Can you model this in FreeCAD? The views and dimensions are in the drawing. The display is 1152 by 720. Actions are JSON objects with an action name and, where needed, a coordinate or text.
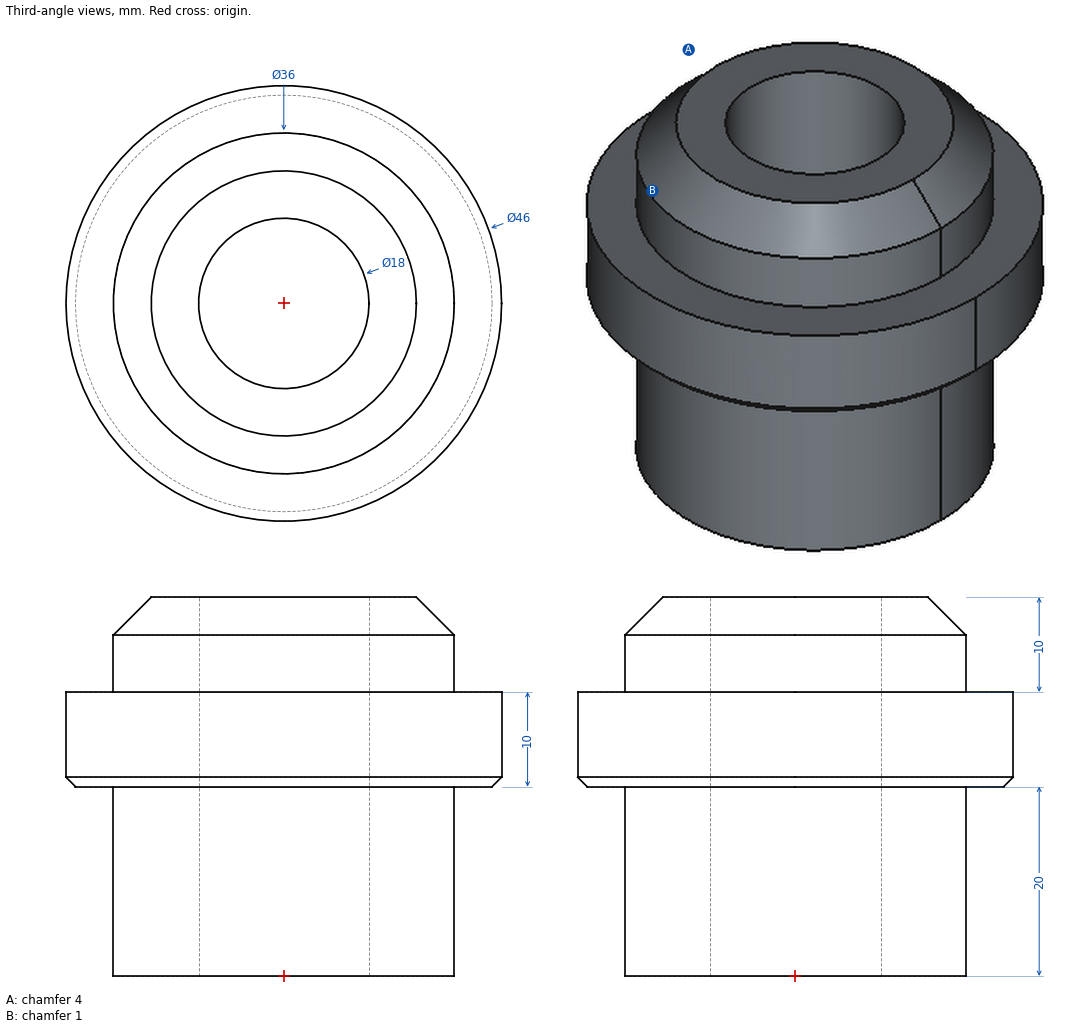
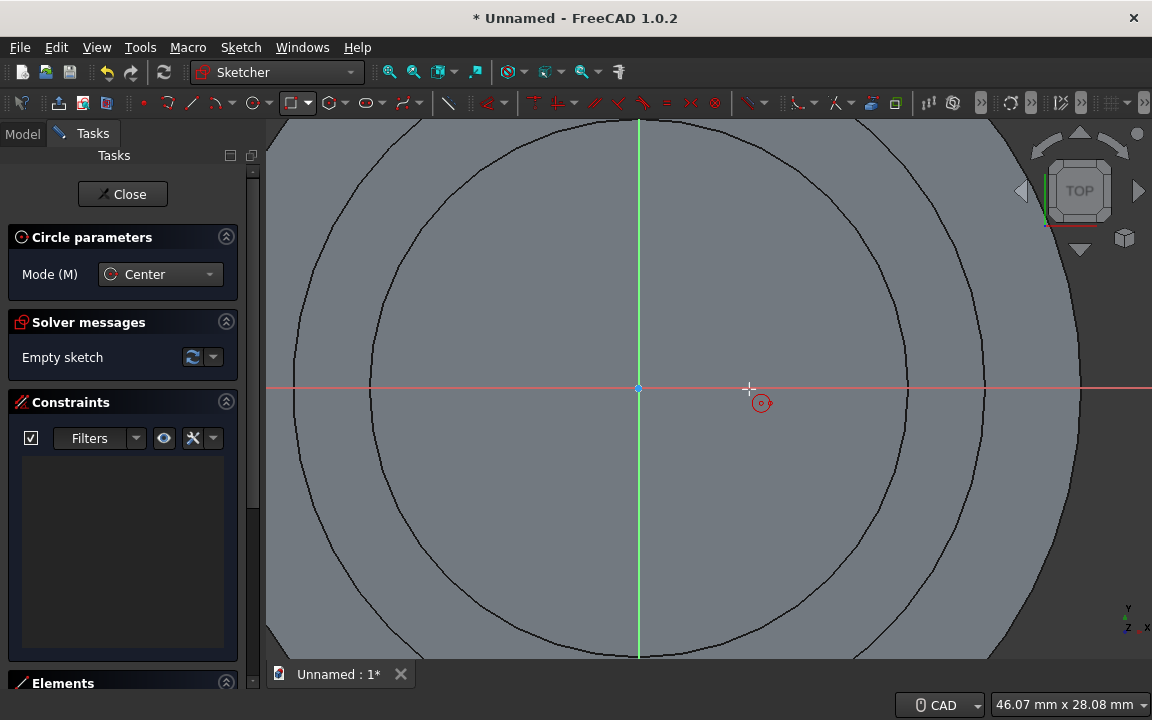
{"action": "left_click", "coordinate": [639, 388]}
{"action": "left_click", "coordinate": [761, 266]}
{"action": "key", "text": "Escape"}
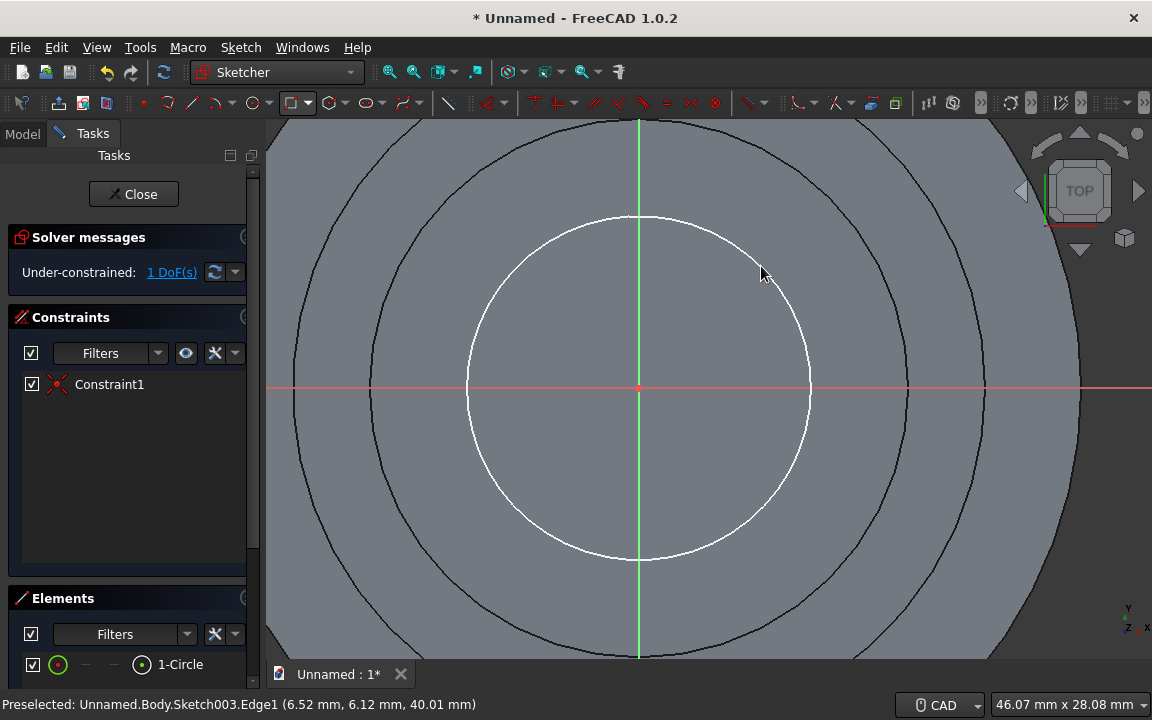
{"action": "left_click", "coordinate": [488, 104]}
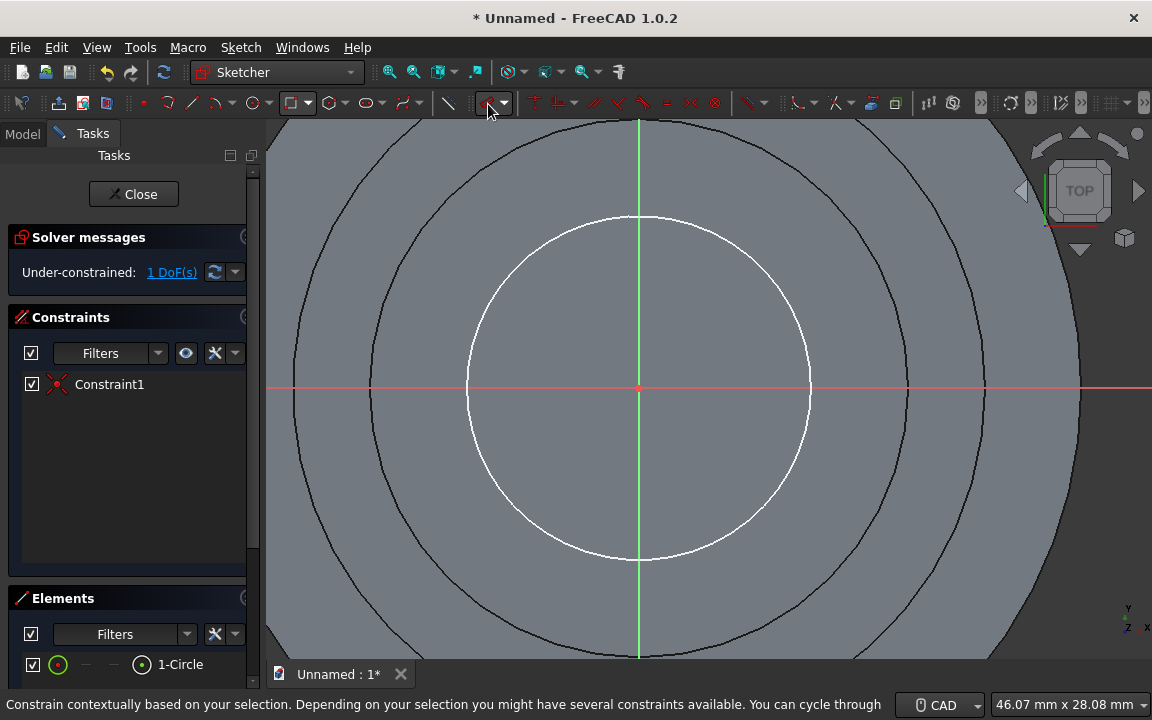
{"action": "left_click", "coordinate": [760, 266]}
{"action": "left_click", "coordinate": [783, 243]}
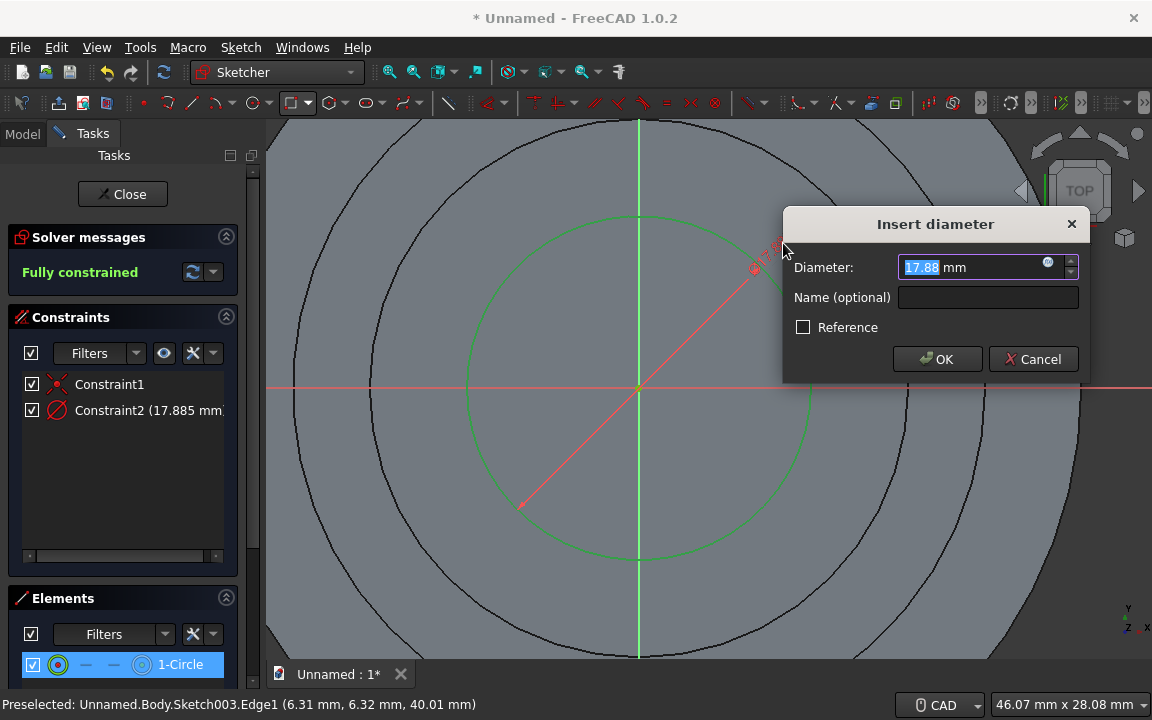
{"action": "type", "text": "18"}
{"action": "key", "text": "Return"}
{"action": "key", "text": "Escape"}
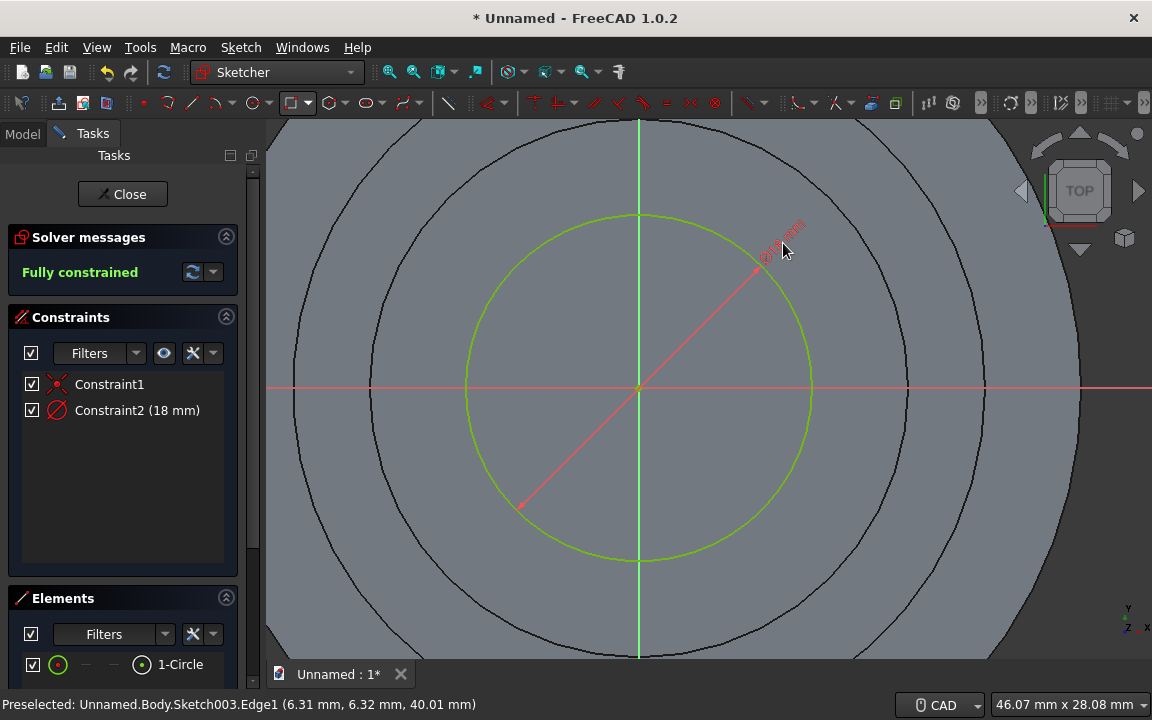
{"action": "left_click", "coordinate": [123, 194]}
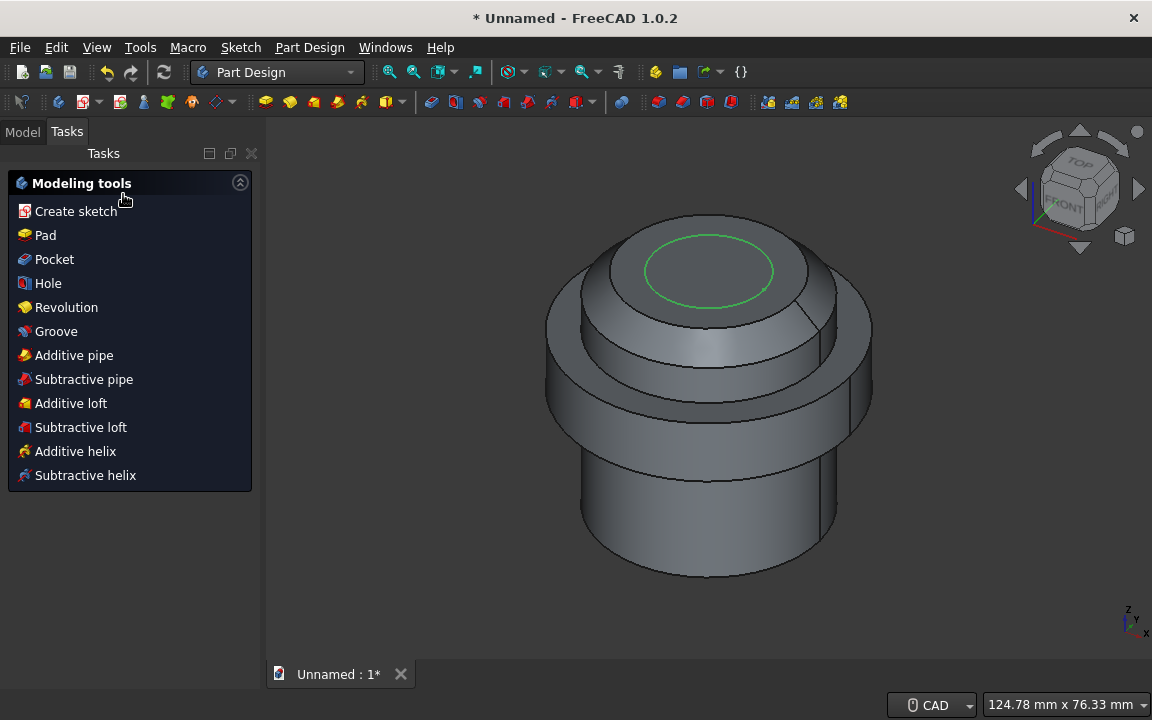
{"action": "left_click", "coordinate": [432, 102]}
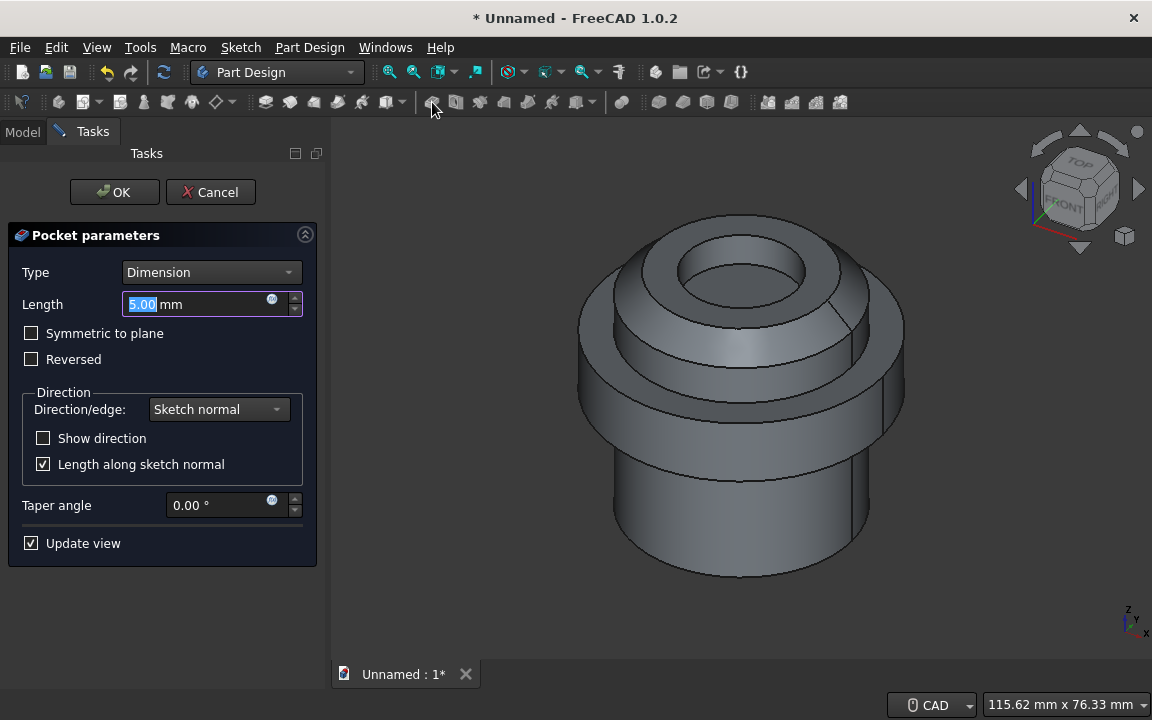
{"action": "left_click", "coordinate": [212, 272]}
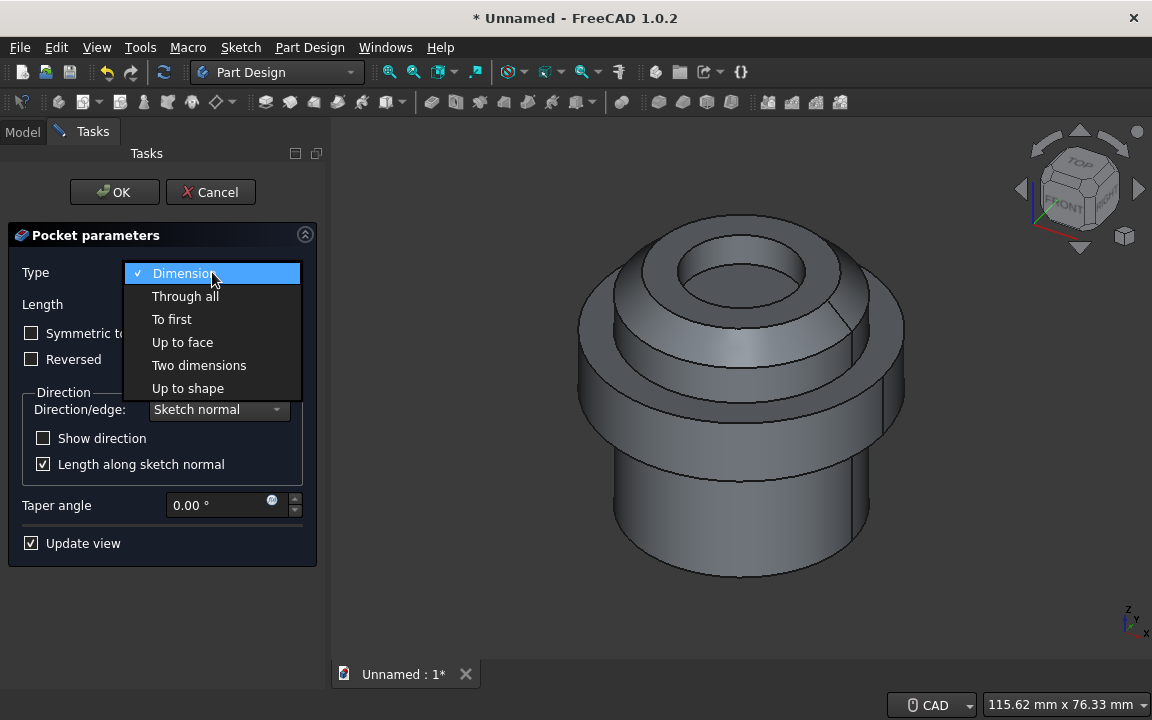
{"action": "left_click", "coordinate": [212, 296]}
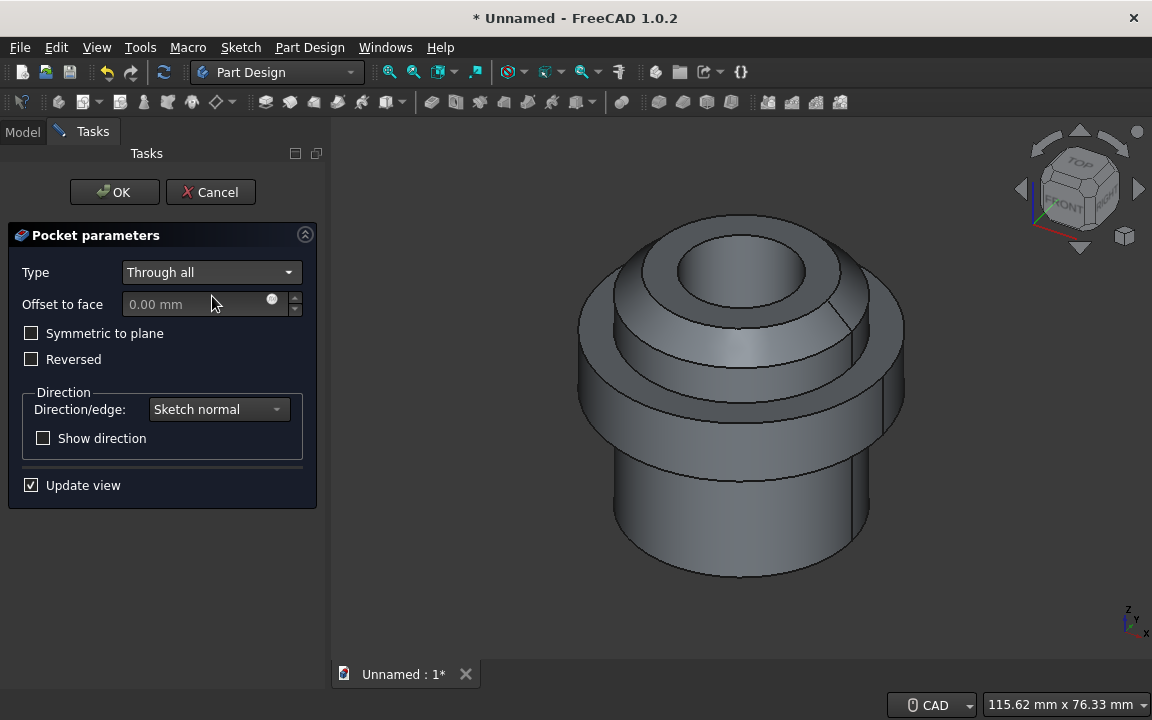
{"action": "left_click", "coordinate": [115, 192]}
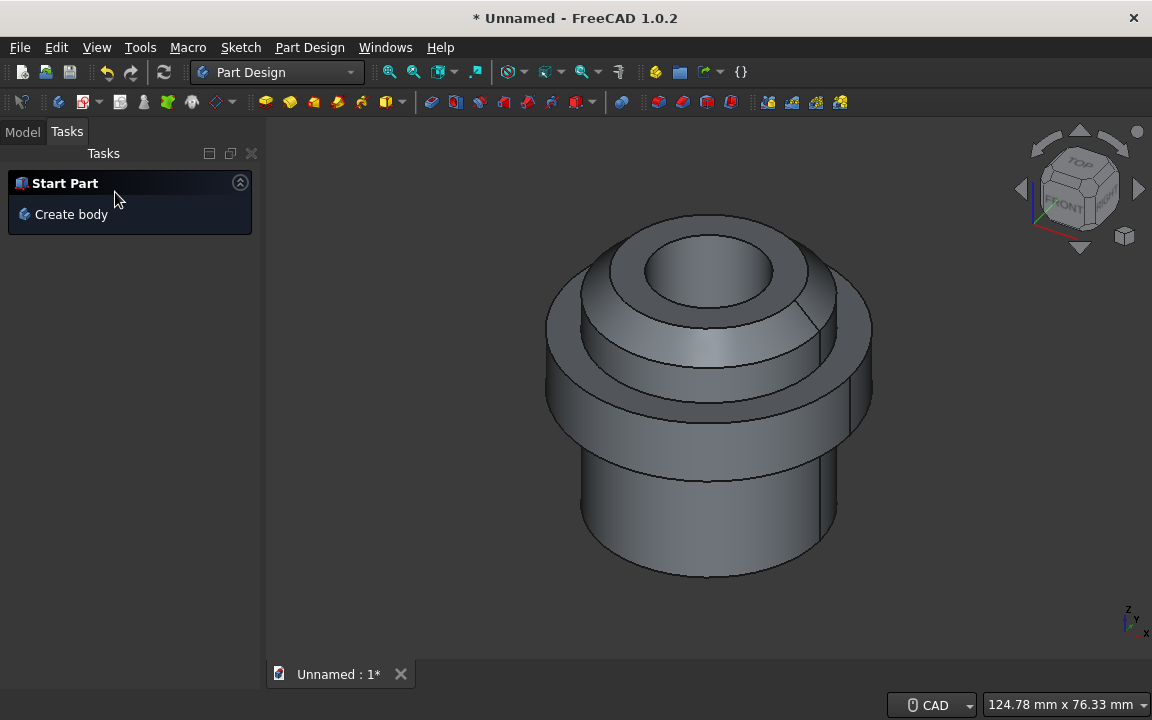
{"action": "key", "text": "0"}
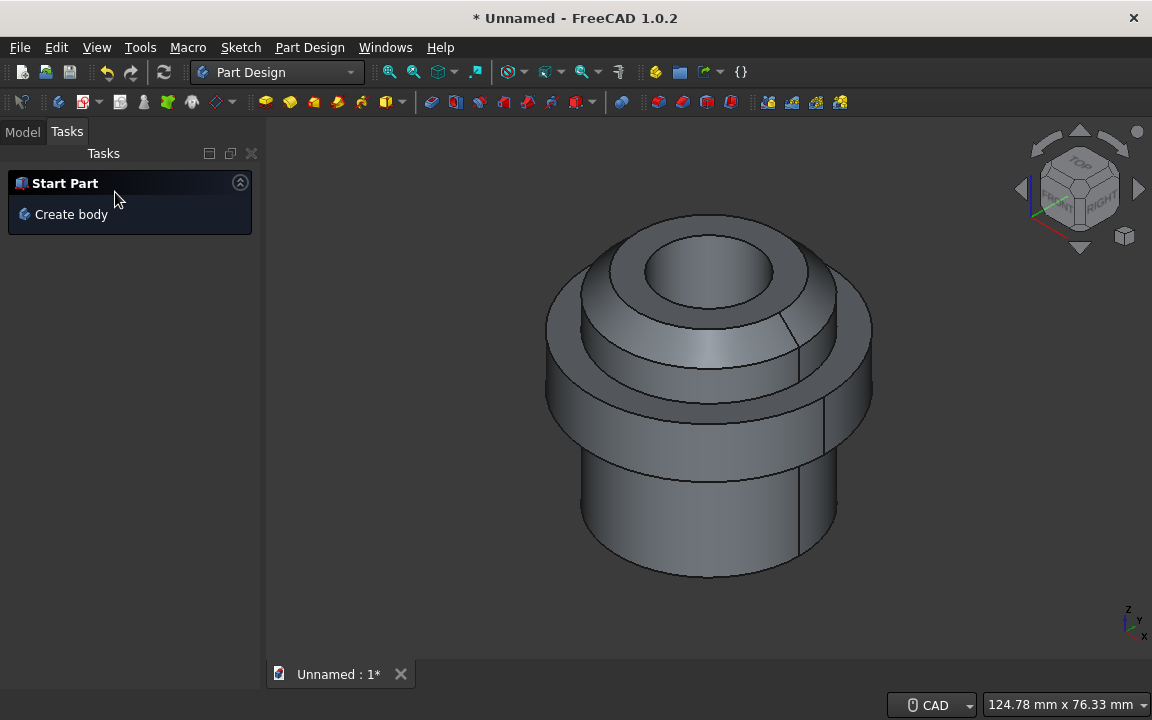
{"action": "key", "text": "2"}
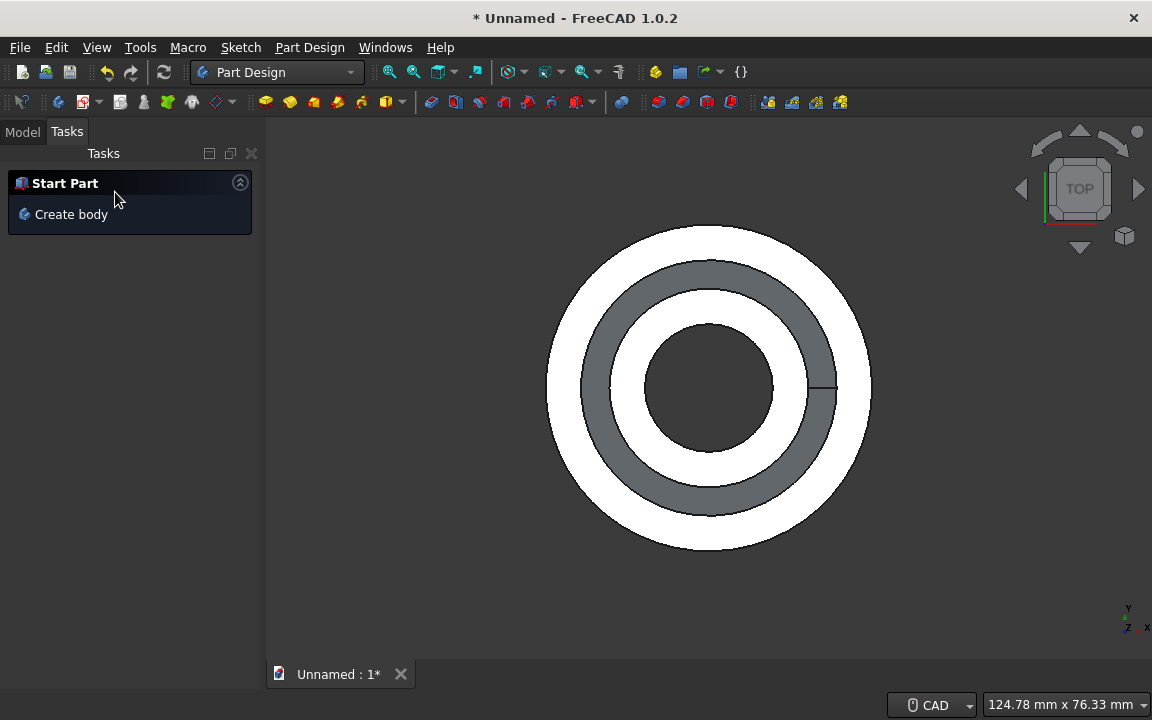
{"action": "key", "text": "1"}